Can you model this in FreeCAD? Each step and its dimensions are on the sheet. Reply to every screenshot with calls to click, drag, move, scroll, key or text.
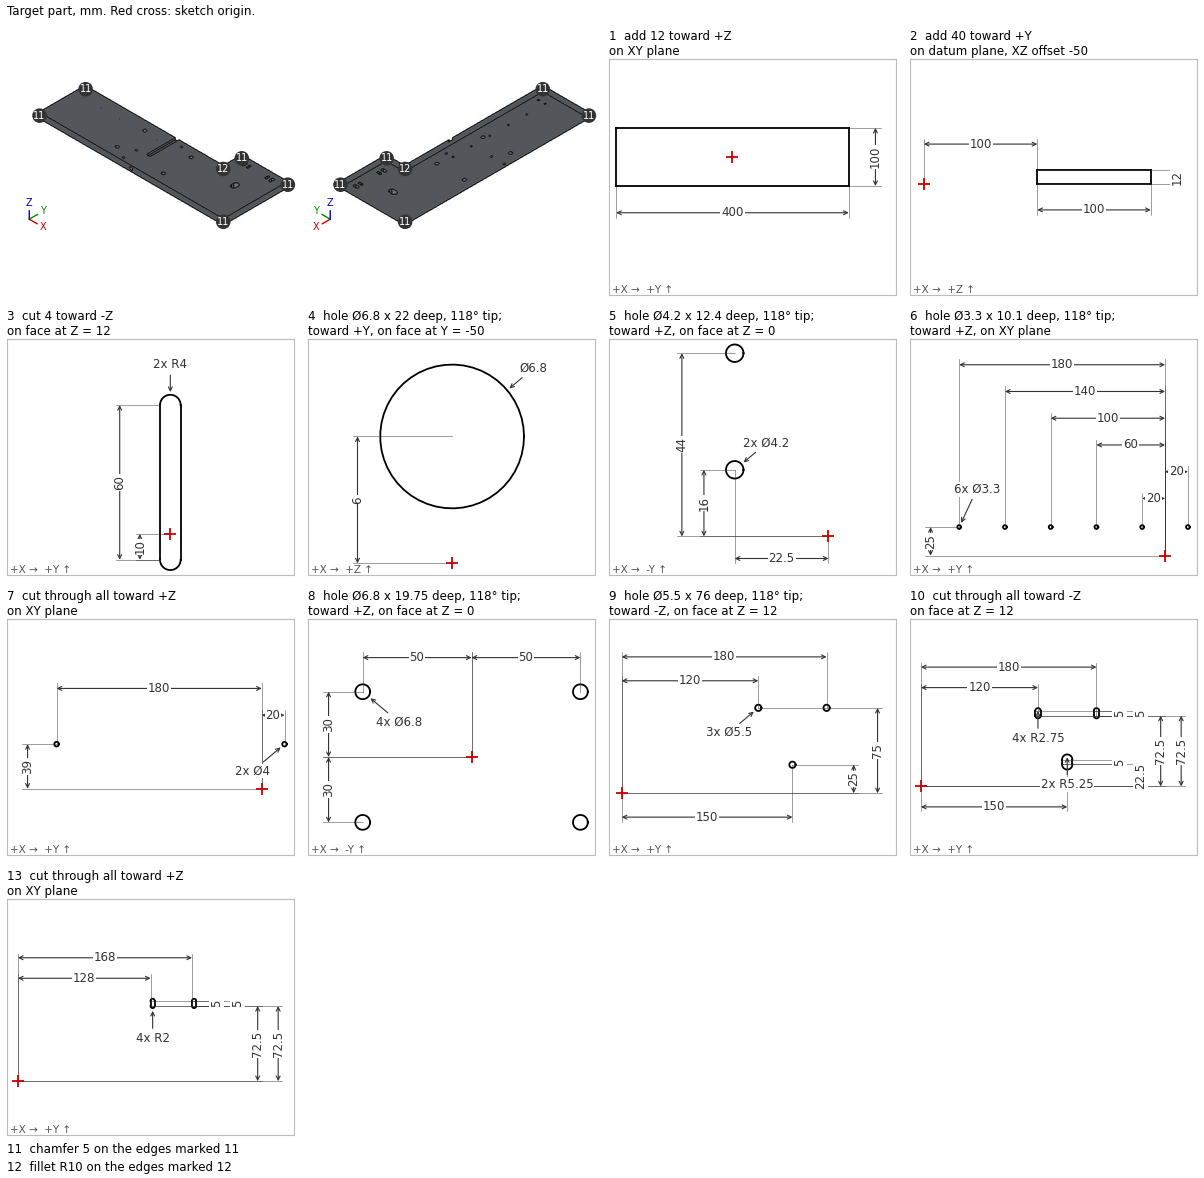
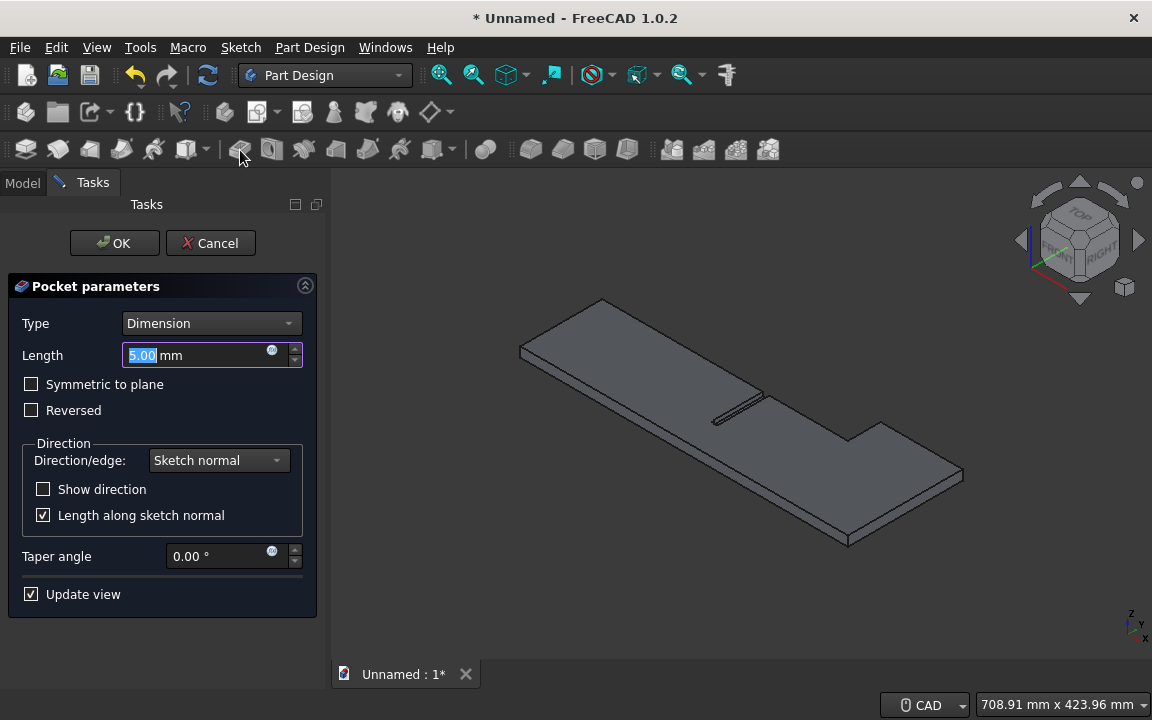
text(4)
key(Tab)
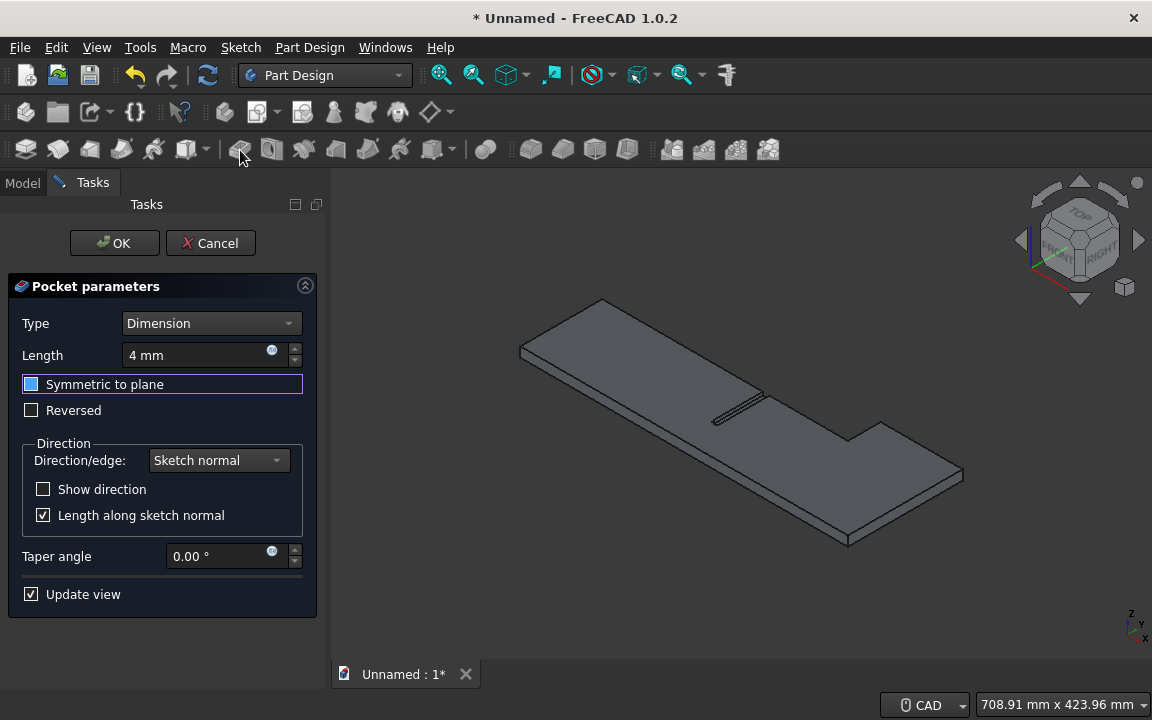
click(115, 243)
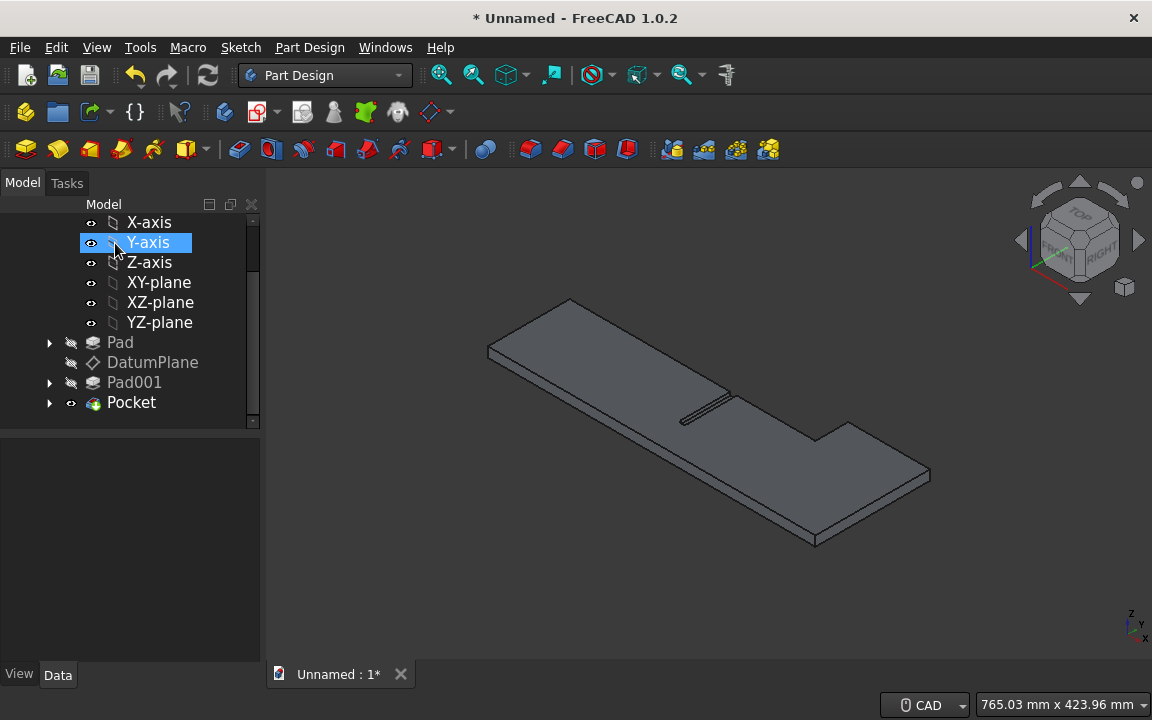
scroll(792, 527, up, 3)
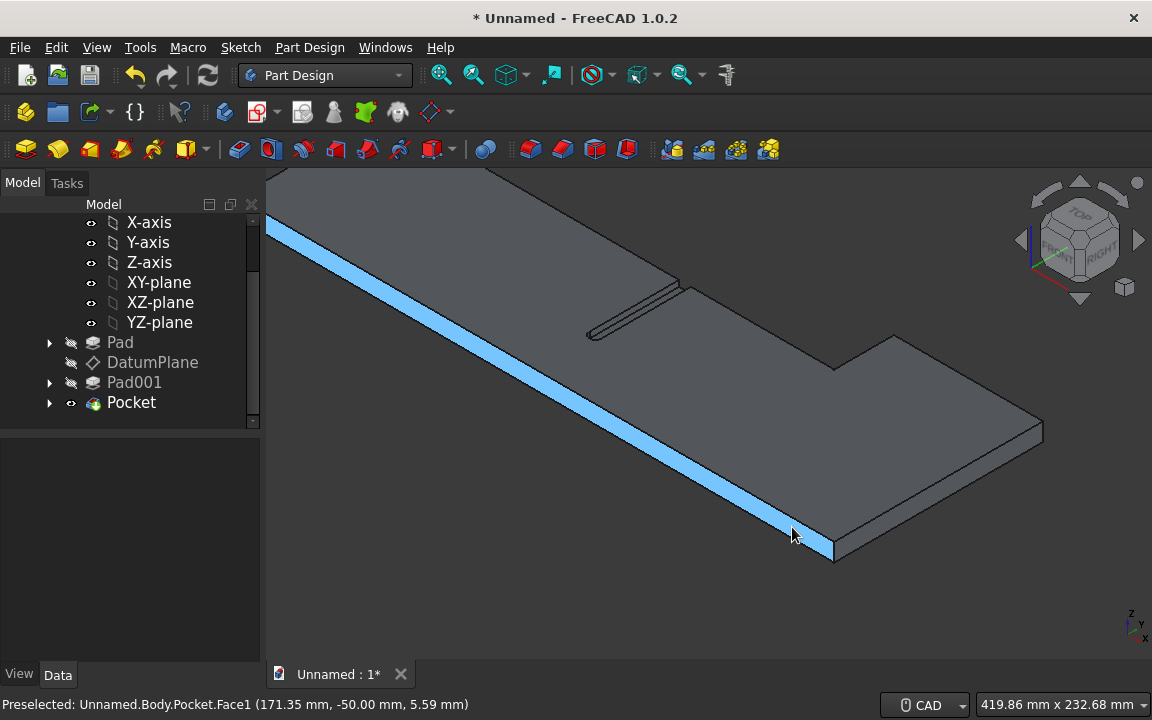
click(792, 527)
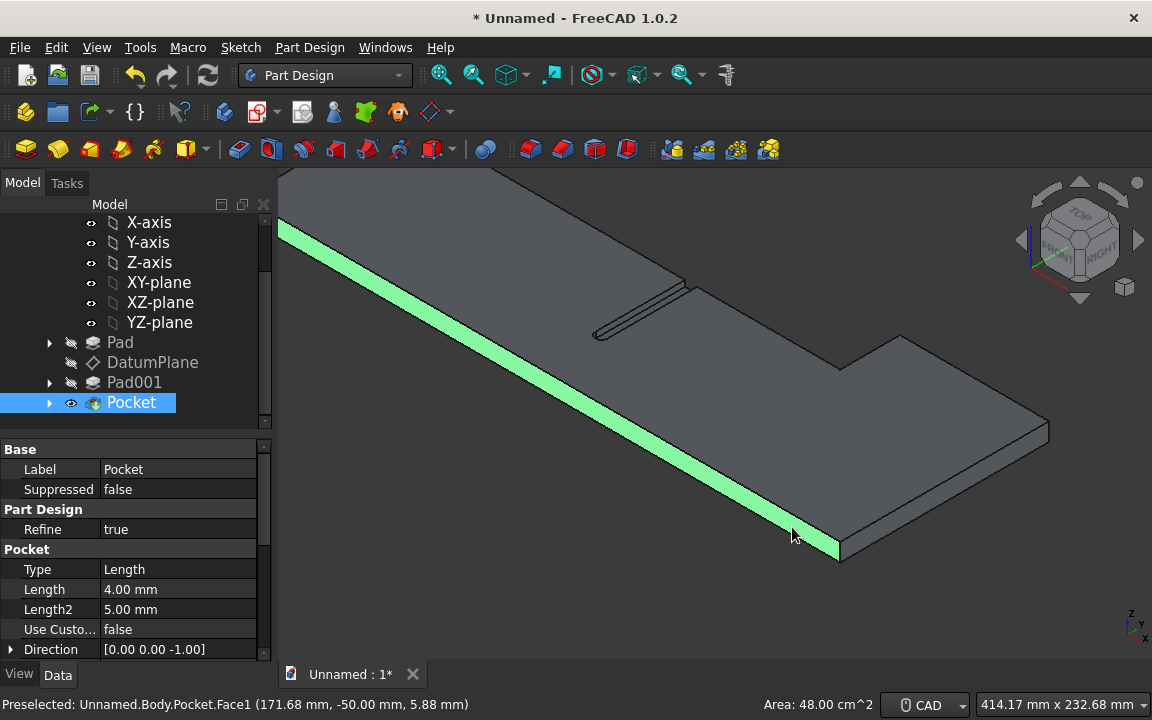
click(258, 112)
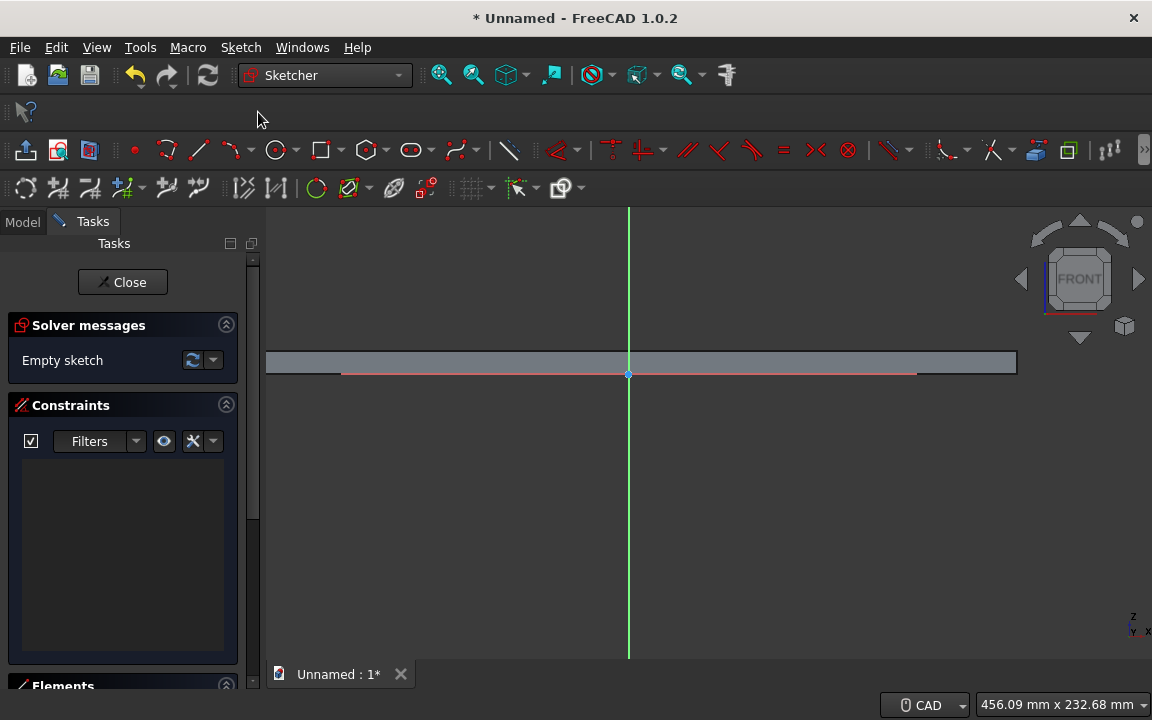
scroll(628, 361, up, 14)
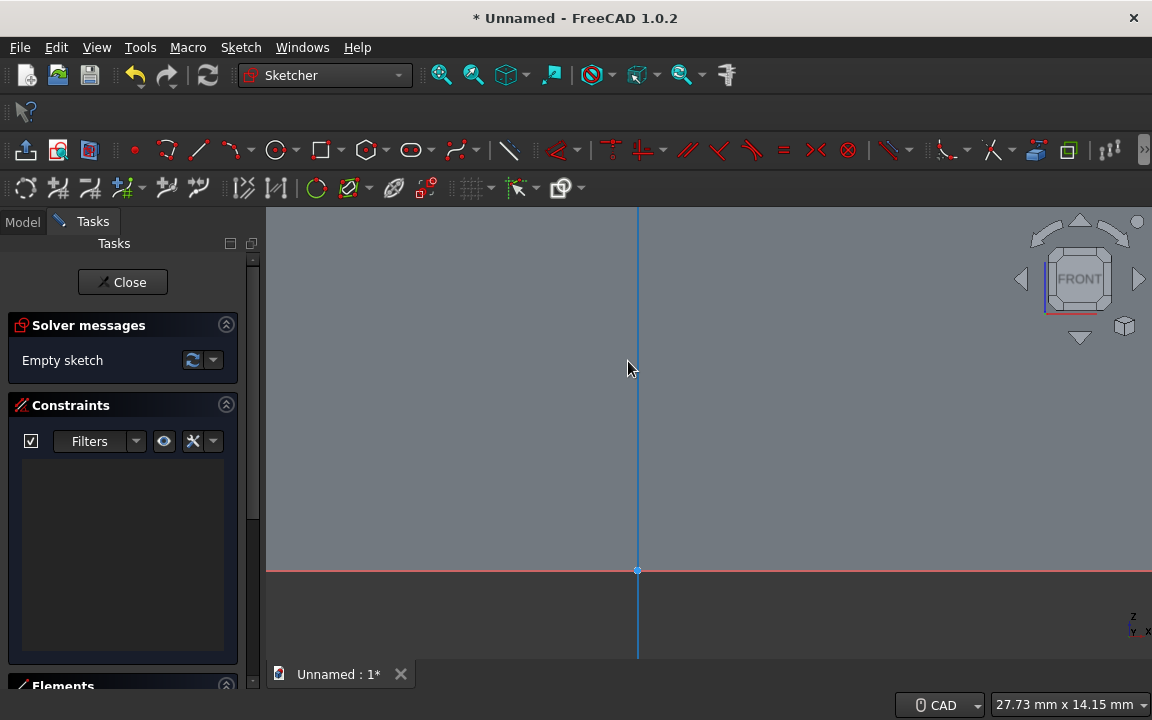
click(276, 150)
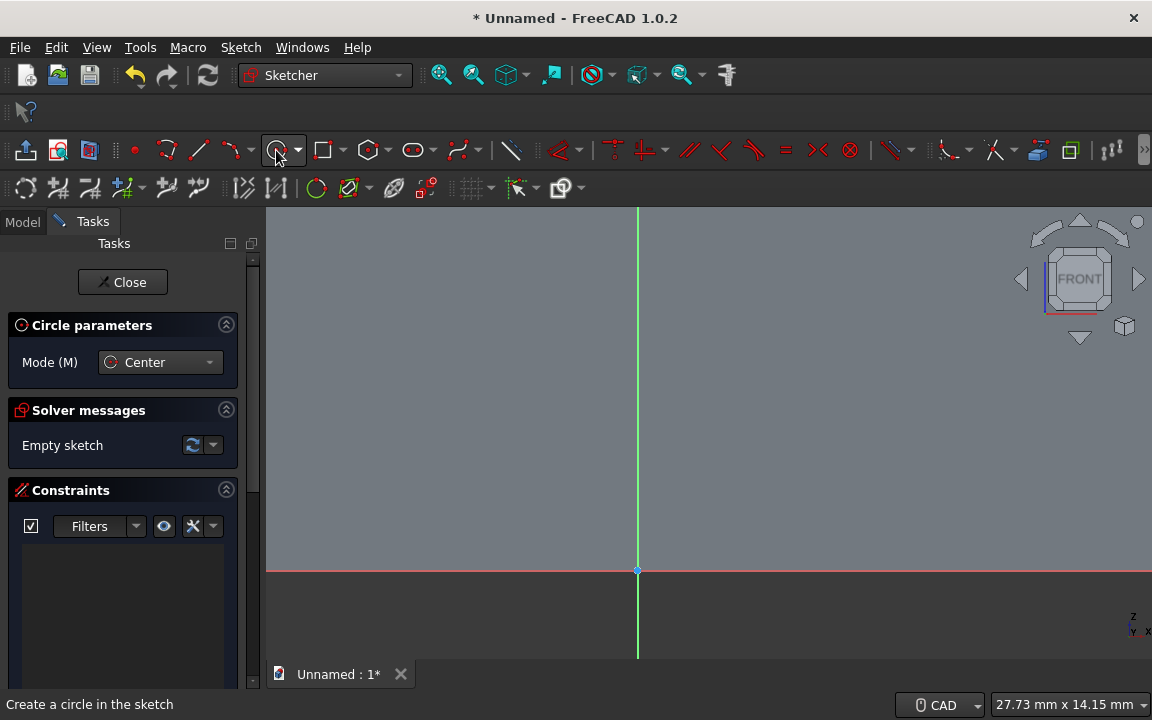
click(638, 379)
move(714, 302)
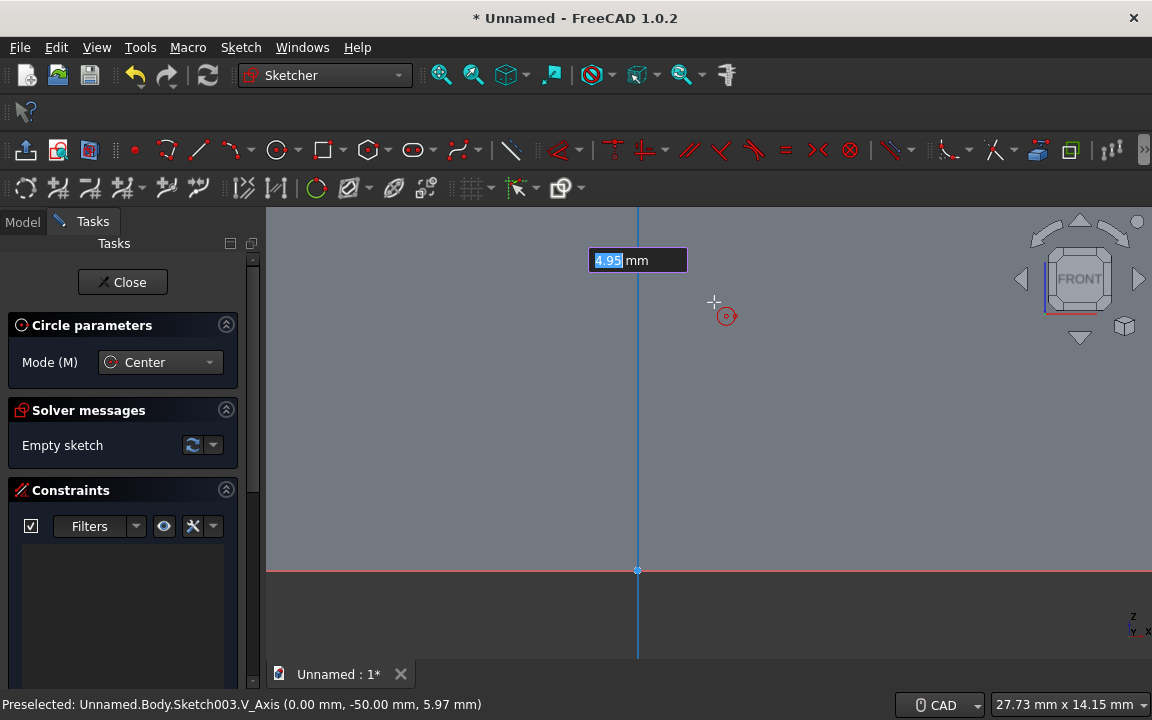
text(6.8)
key(Return)
key(Escape)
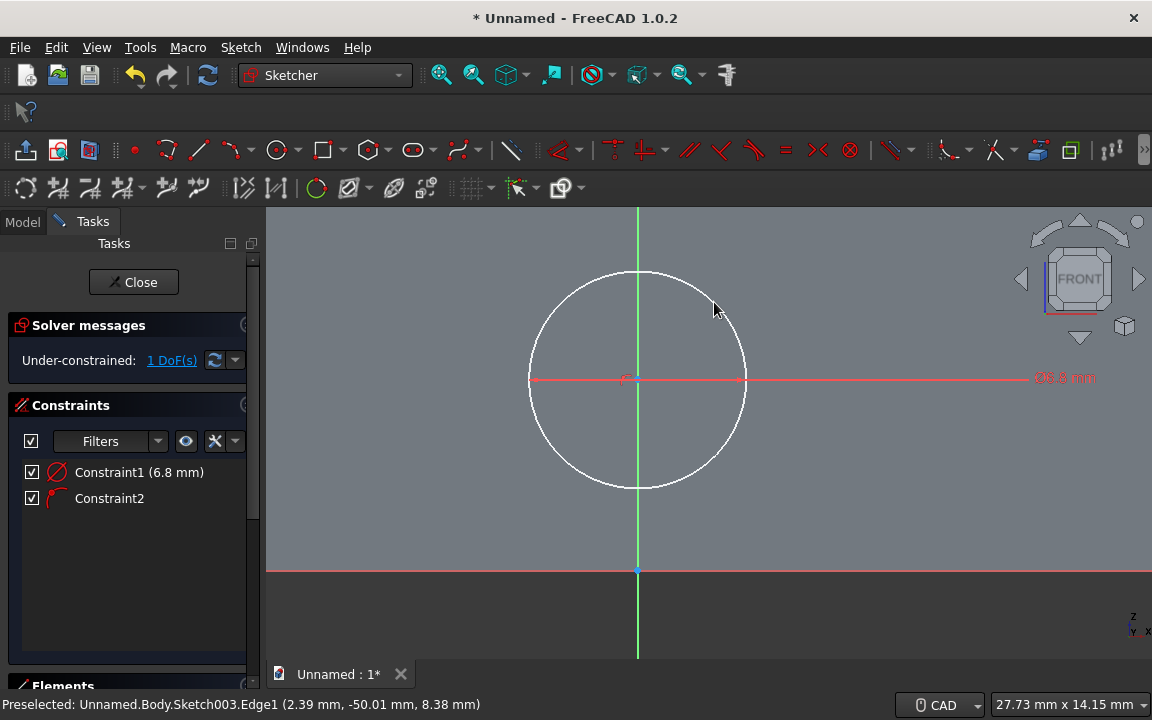
click(558, 150)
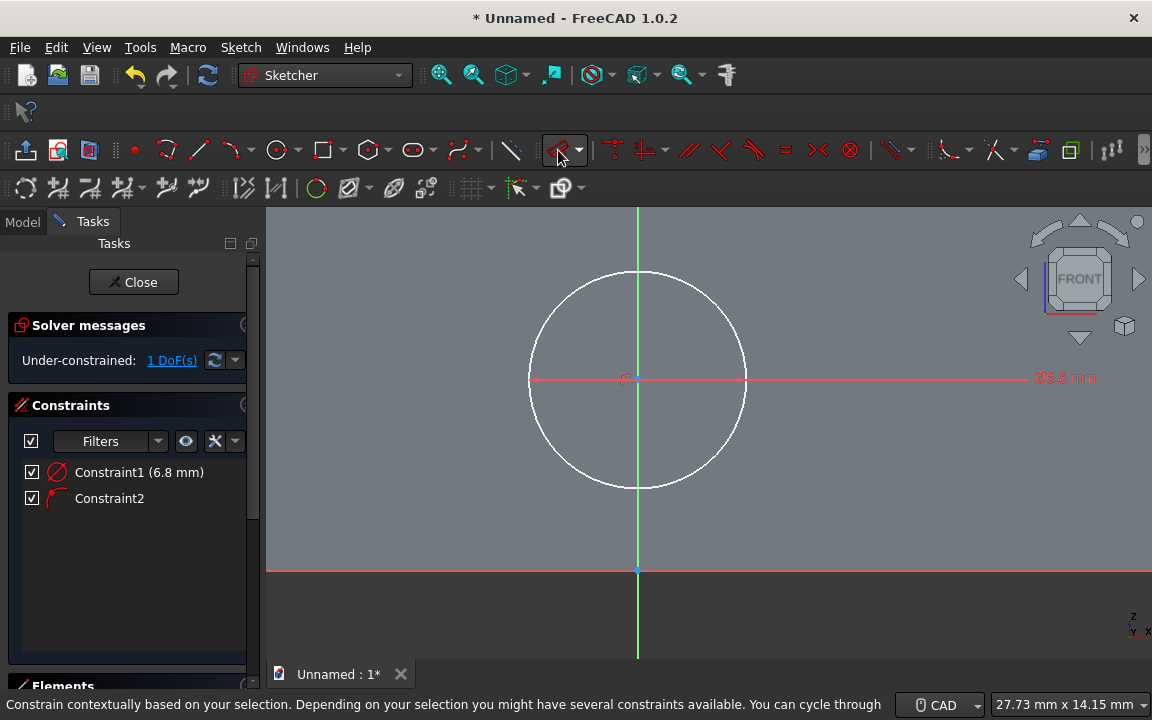
click(638, 380)
click(672, 431)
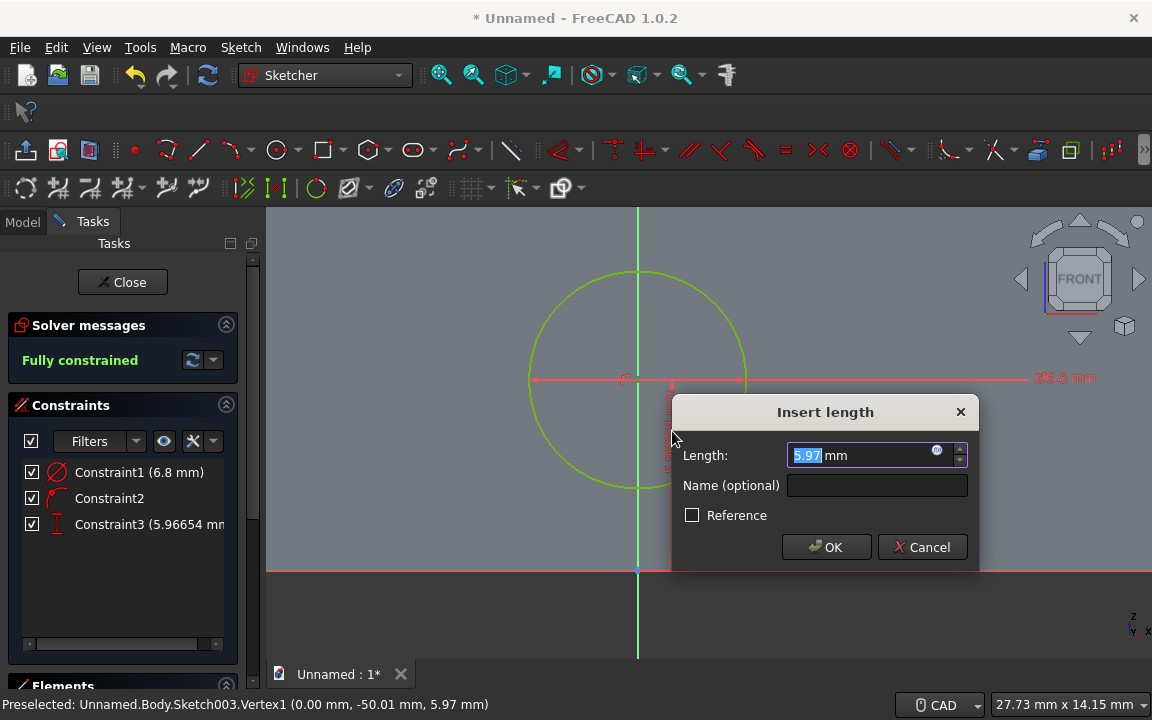
text(6)
key(Return)
key(Escape)